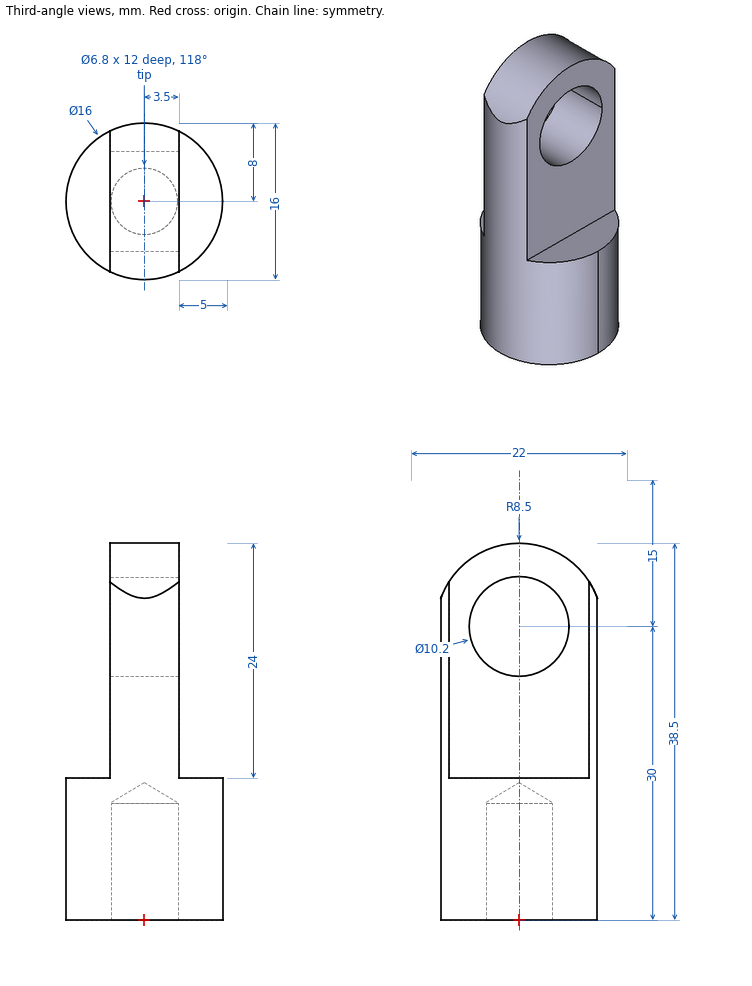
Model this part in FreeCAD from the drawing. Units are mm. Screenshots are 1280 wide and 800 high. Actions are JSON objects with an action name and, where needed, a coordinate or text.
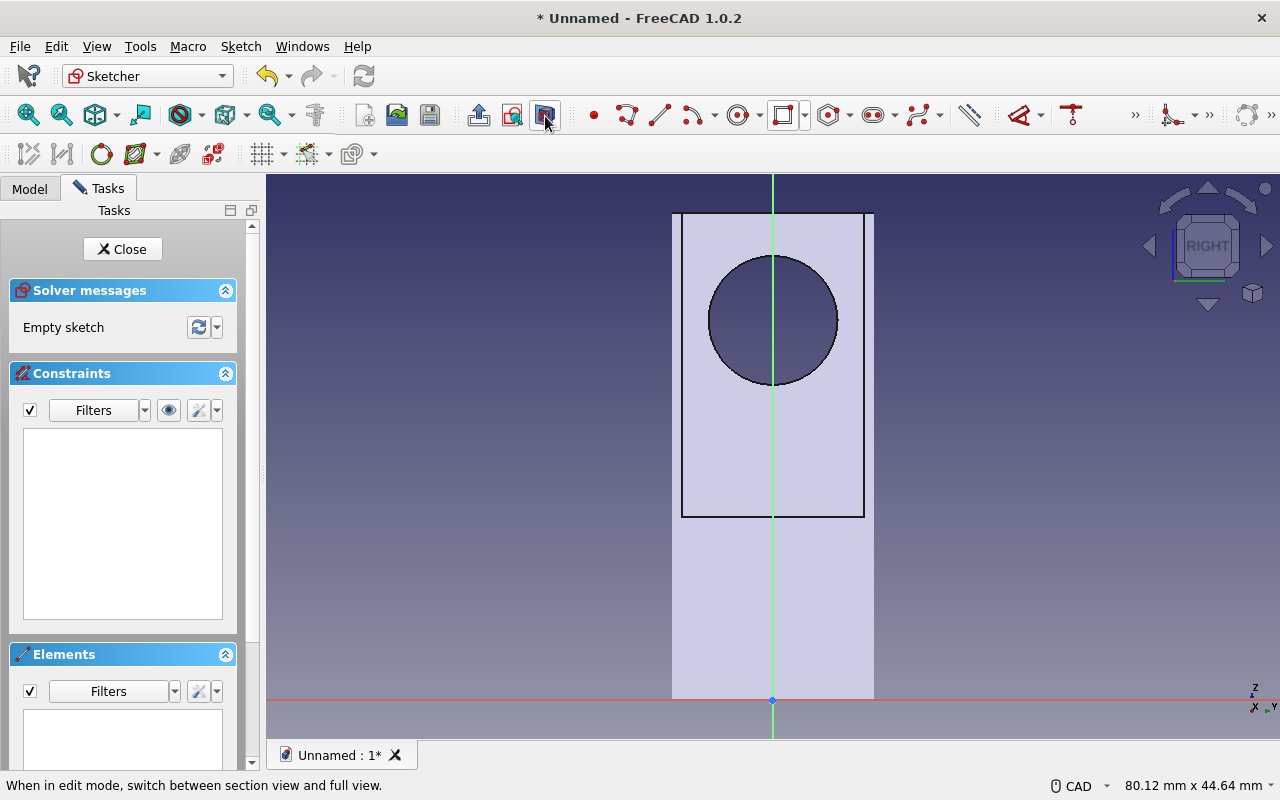
{"action": "scroll", "coordinate": [565, 540], "scroll_direction": "down", "scroll_amount": 2}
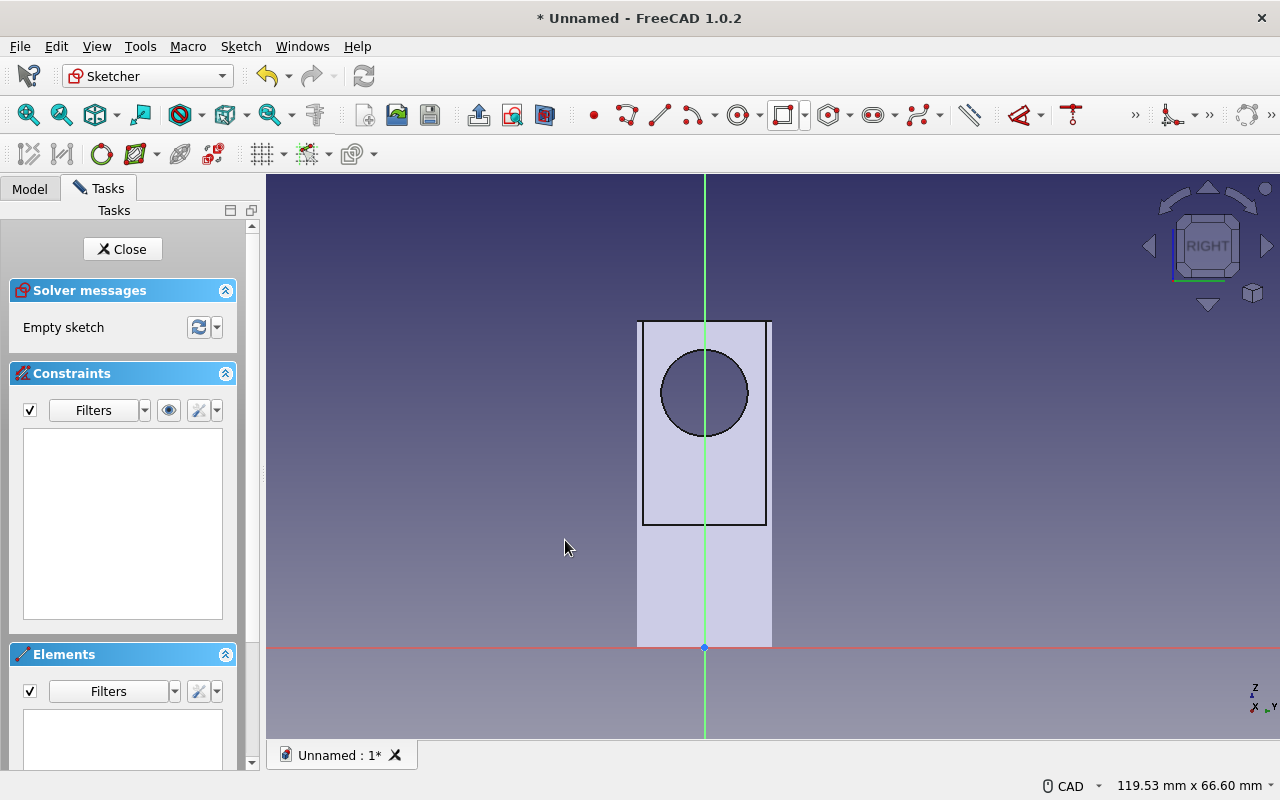
{"action": "key", "text": "g m"}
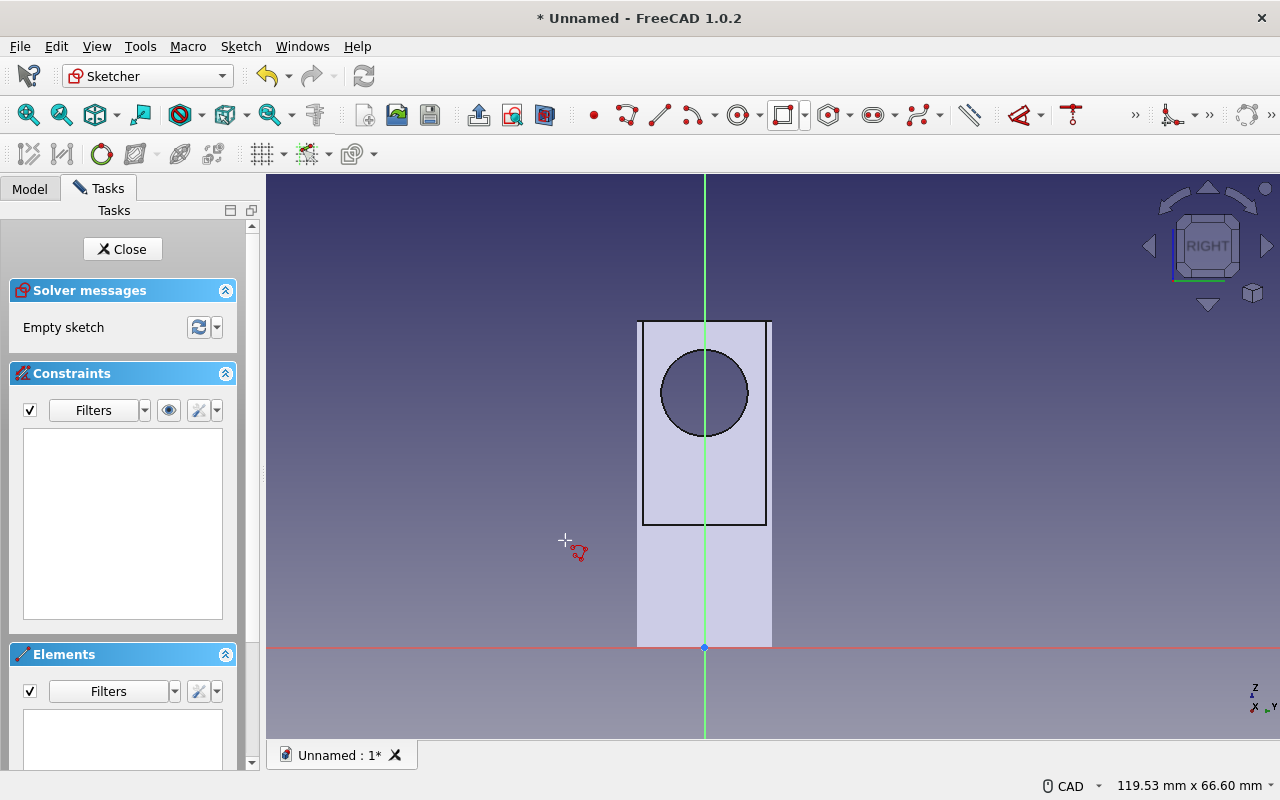
{"action": "left_click", "coordinate": [777, 393]}
{"action": "left_click", "coordinate": [798, 393]}
{"action": "left_click", "coordinate": [798, 266]}
{"action": "left_click", "coordinate": [611, 266]}
{"action": "left_click", "coordinate": [611, 393]}
{"action": "left_click", "coordinate": [632, 393]}
{"action": "right_click", "coordinate": [632, 393]}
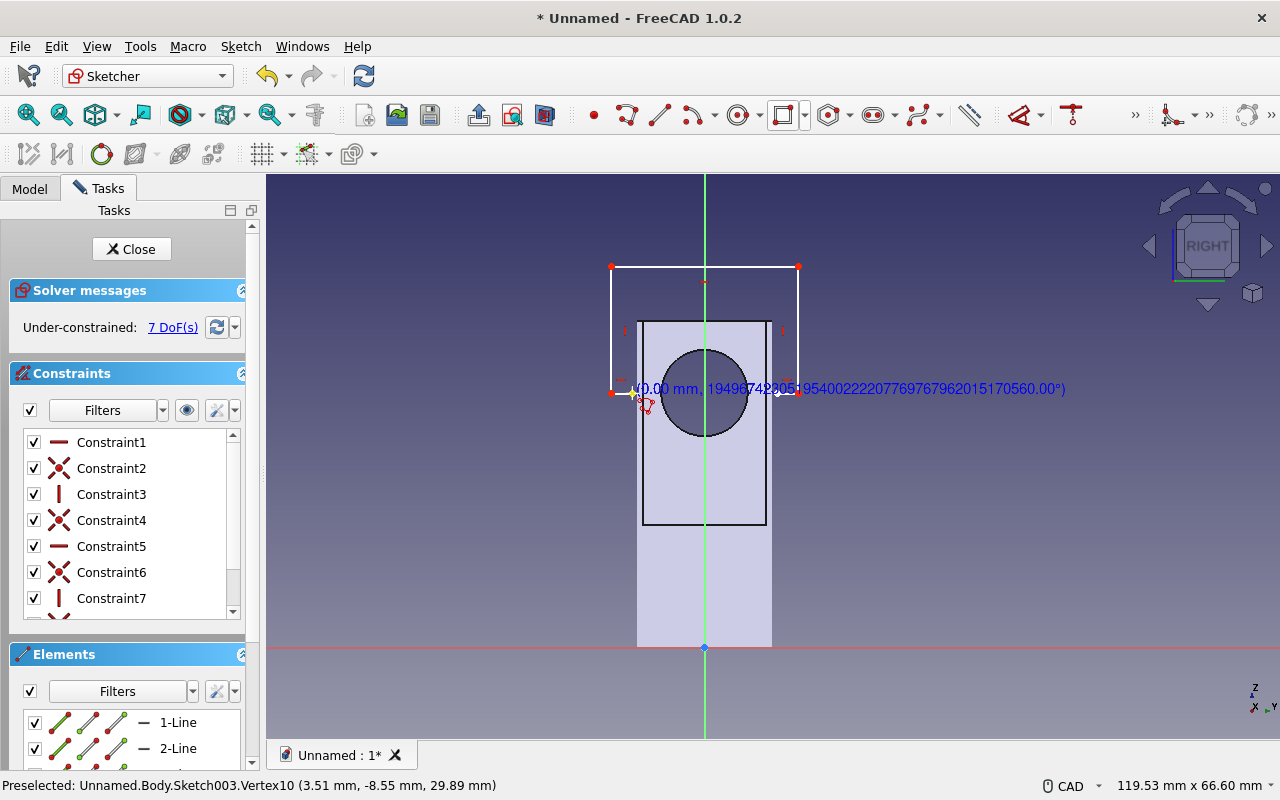
{"action": "key", "text": "g 3 a"}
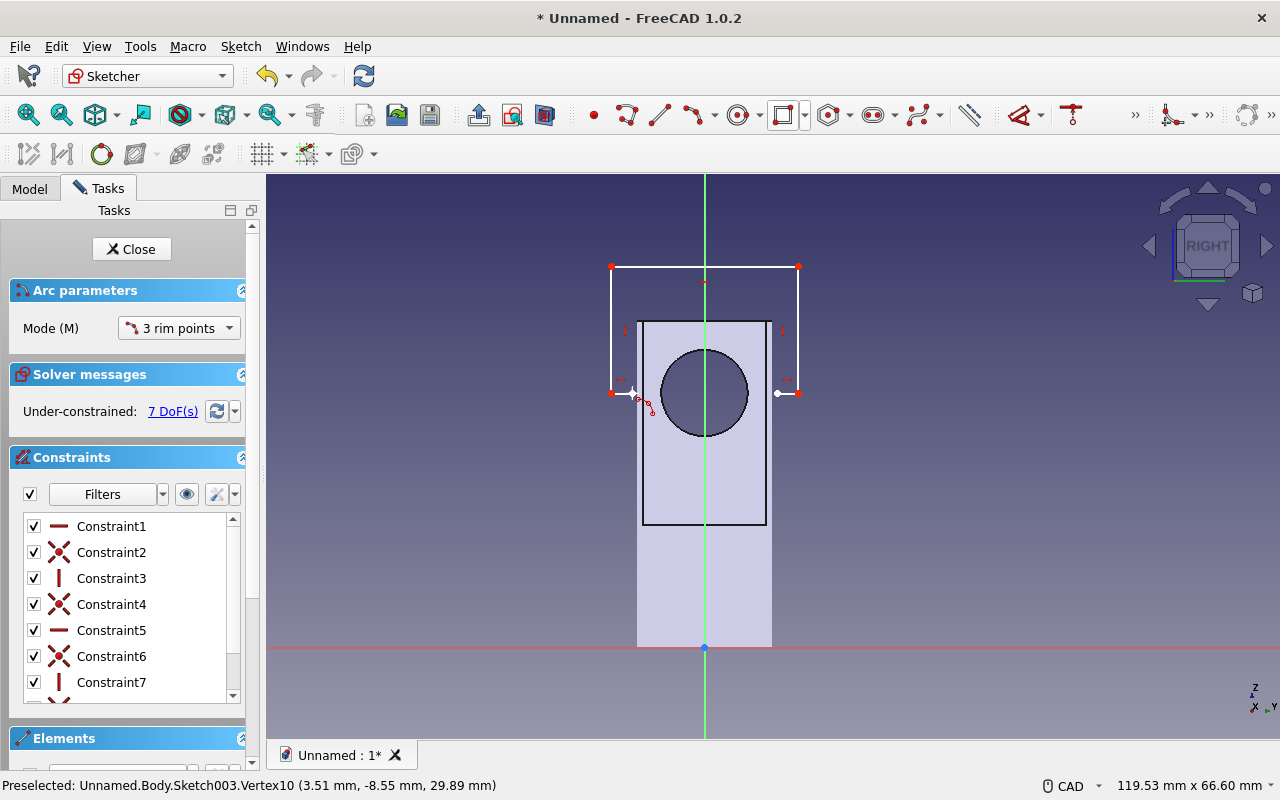
{"action": "scroll", "coordinate": [632, 393], "scroll_direction": "up", "scroll_amount": 3}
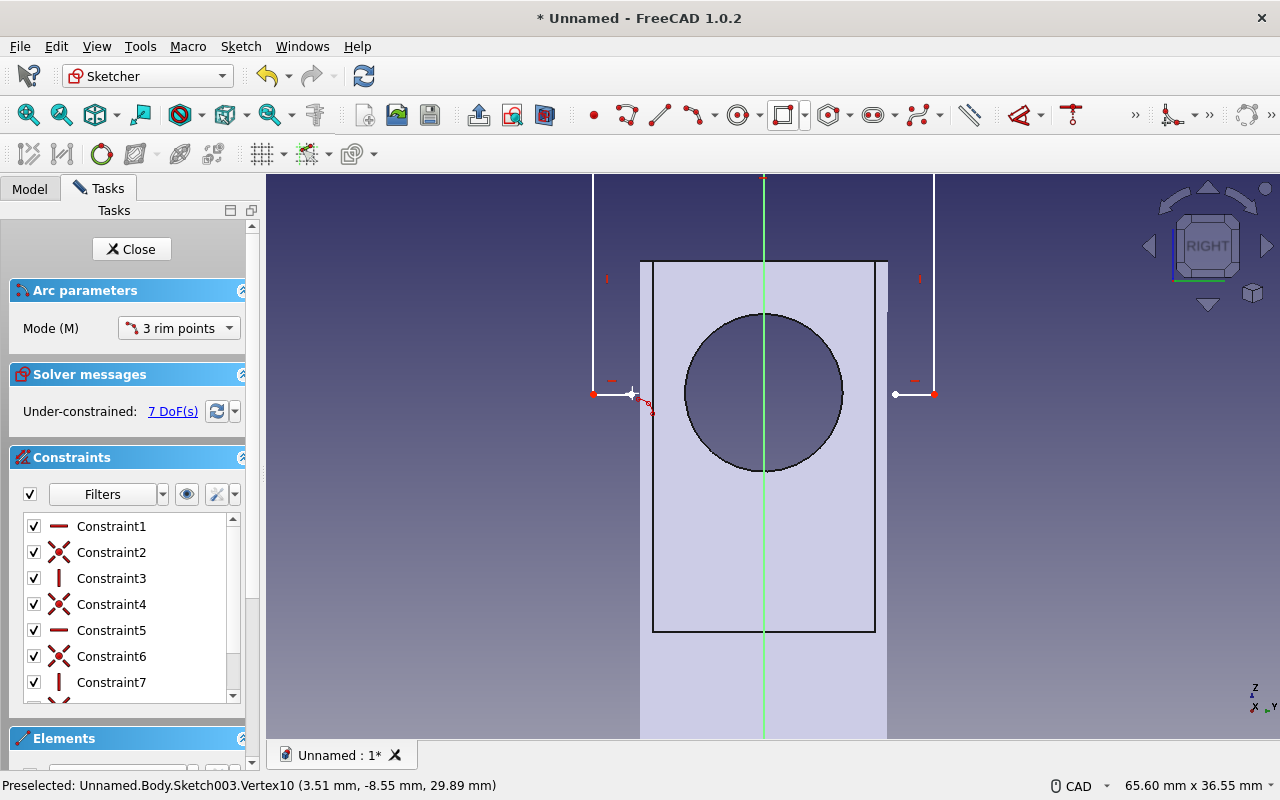
{"action": "left_click", "coordinate": [632, 395]}
{"action": "left_click", "coordinate": [896, 395]}
{"action": "left_click", "coordinate": [804, 268]}
{"action": "key", "text": "Escape"}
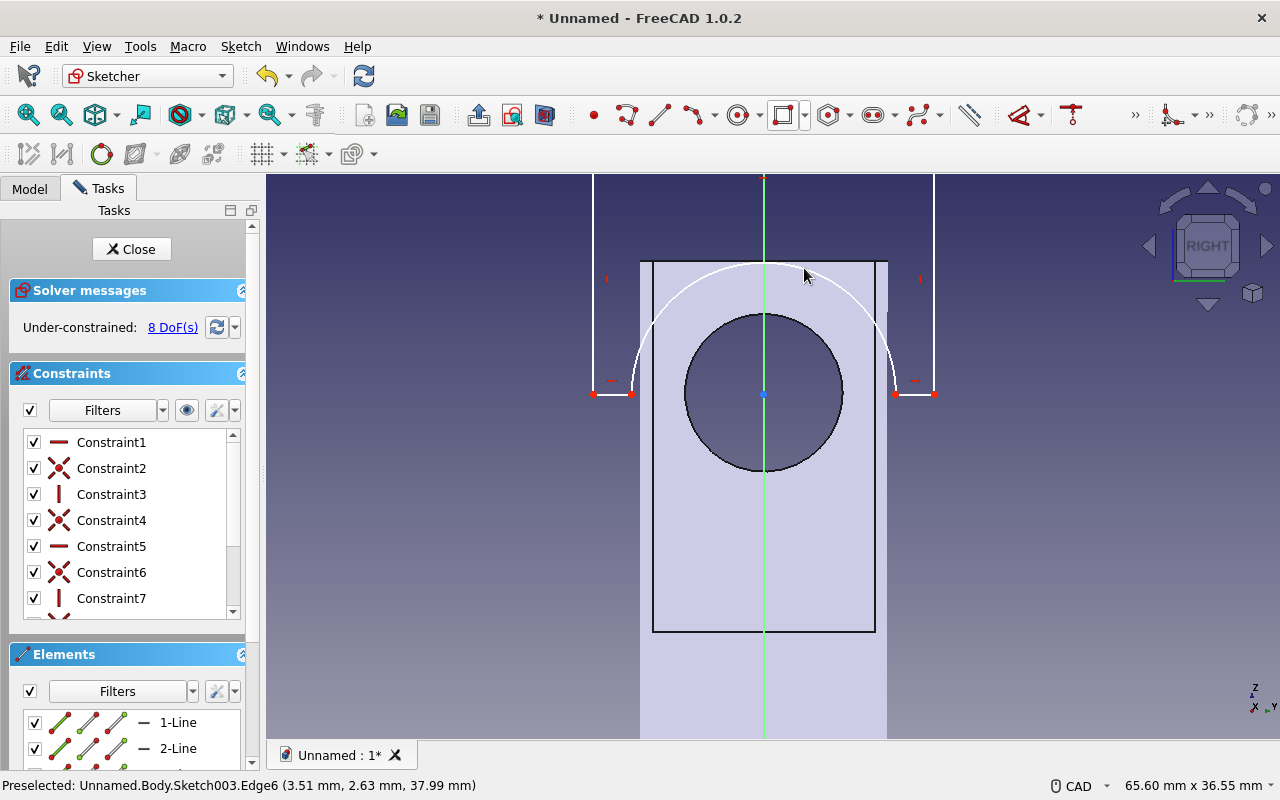
{"action": "left_click", "coordinate": [764, 395]}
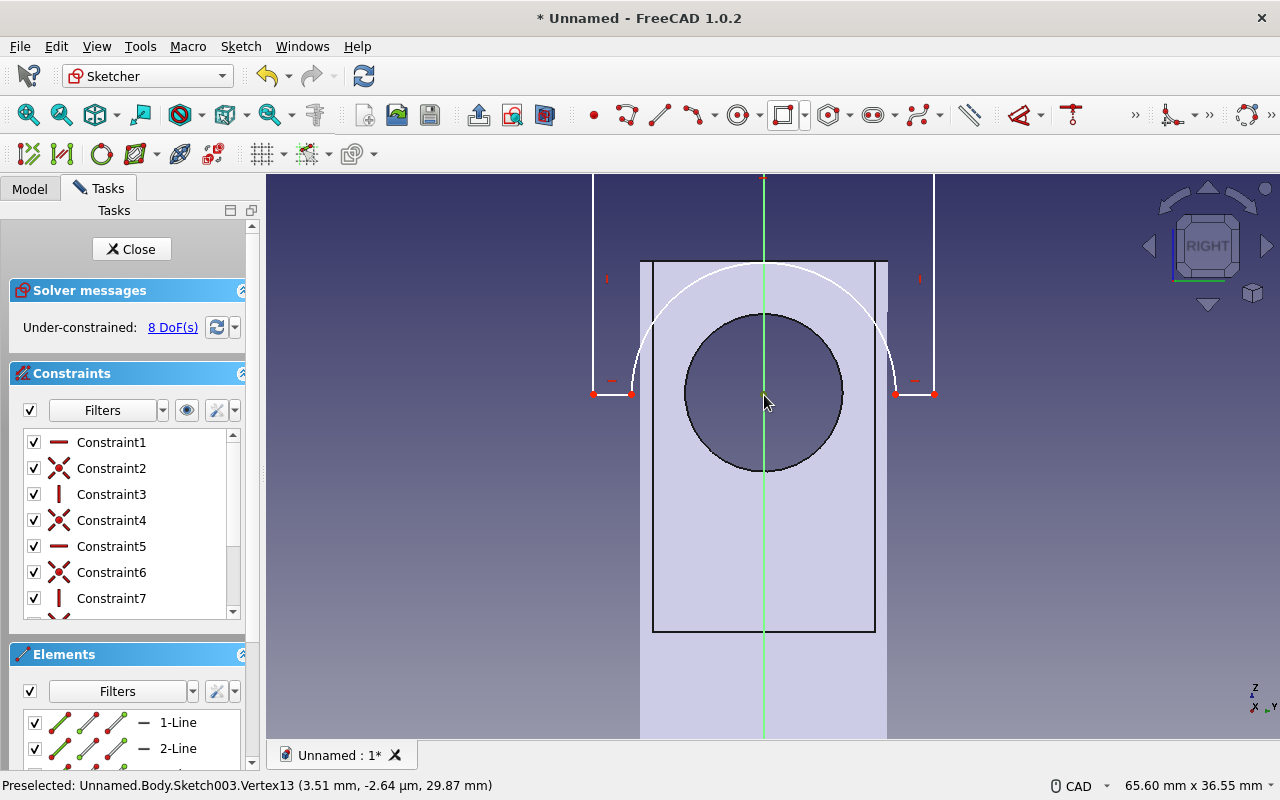
{"action": "left_click", "coordinate": [764, 675]}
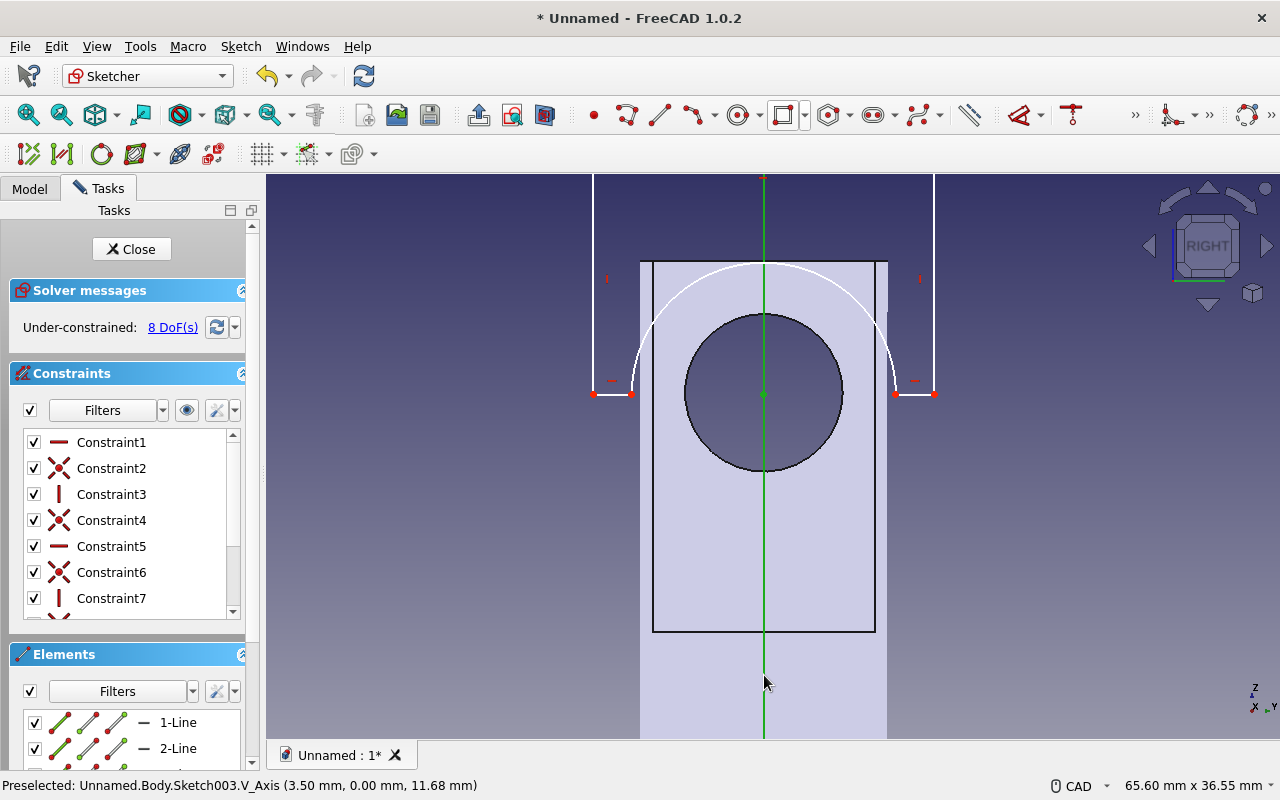
{"action": "key", "text": "c"}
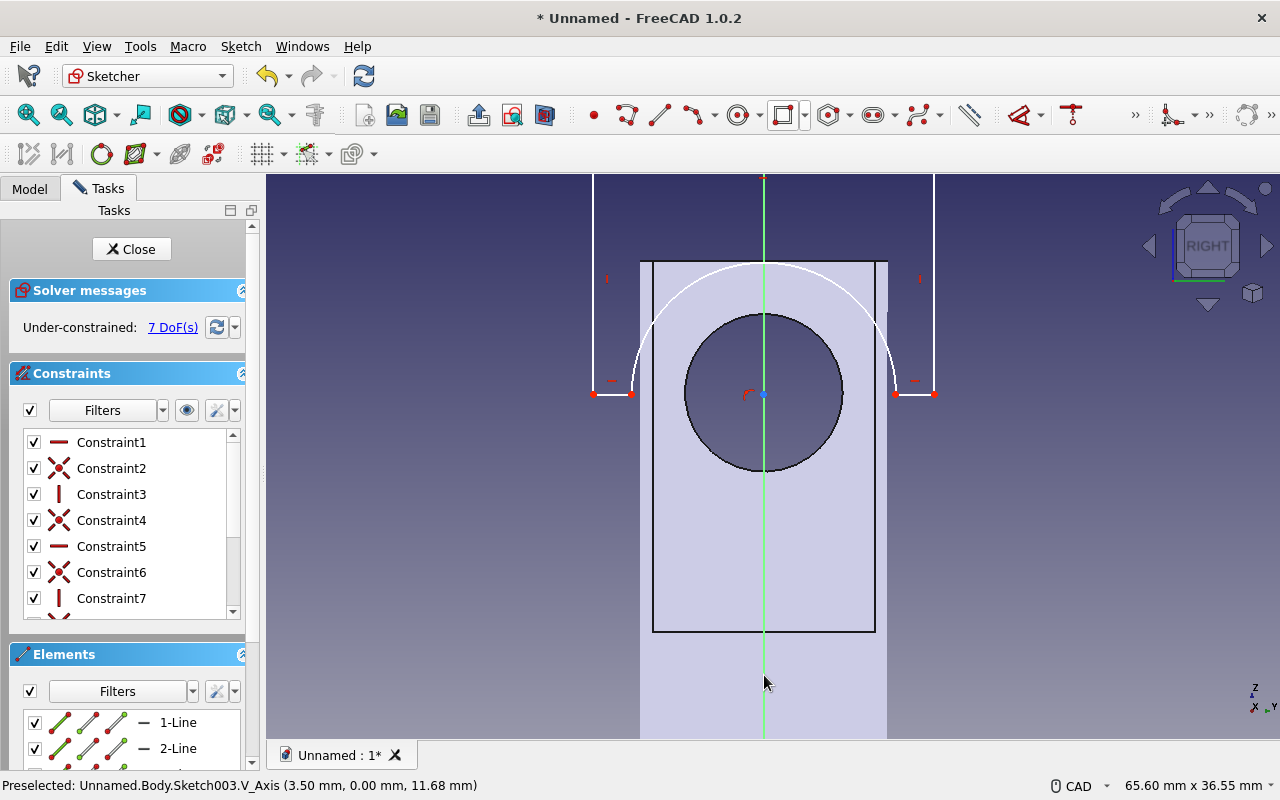
{"action": "left_click", "coordinate": [934, 395]}